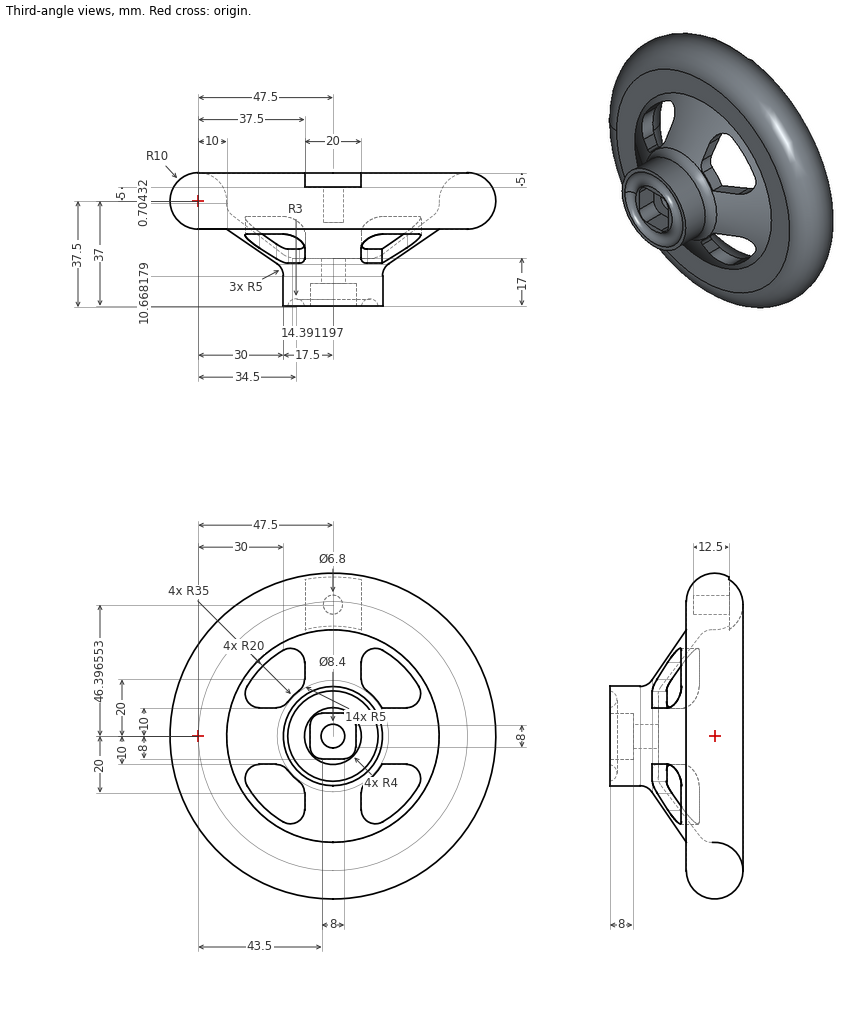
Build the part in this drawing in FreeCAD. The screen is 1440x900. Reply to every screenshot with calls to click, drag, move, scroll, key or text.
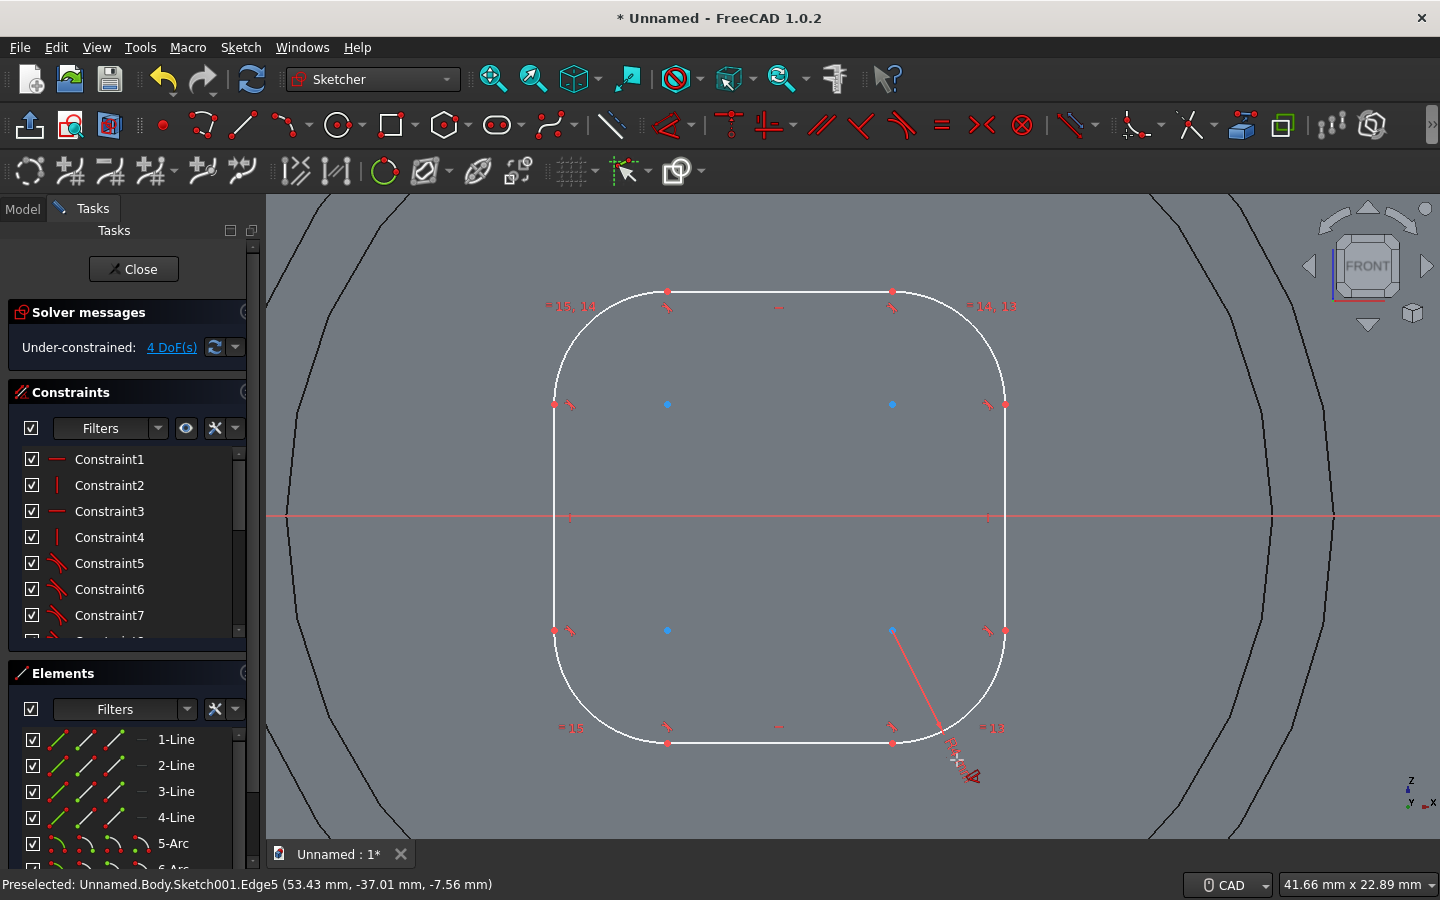
click(735, 743)
click(780, 777)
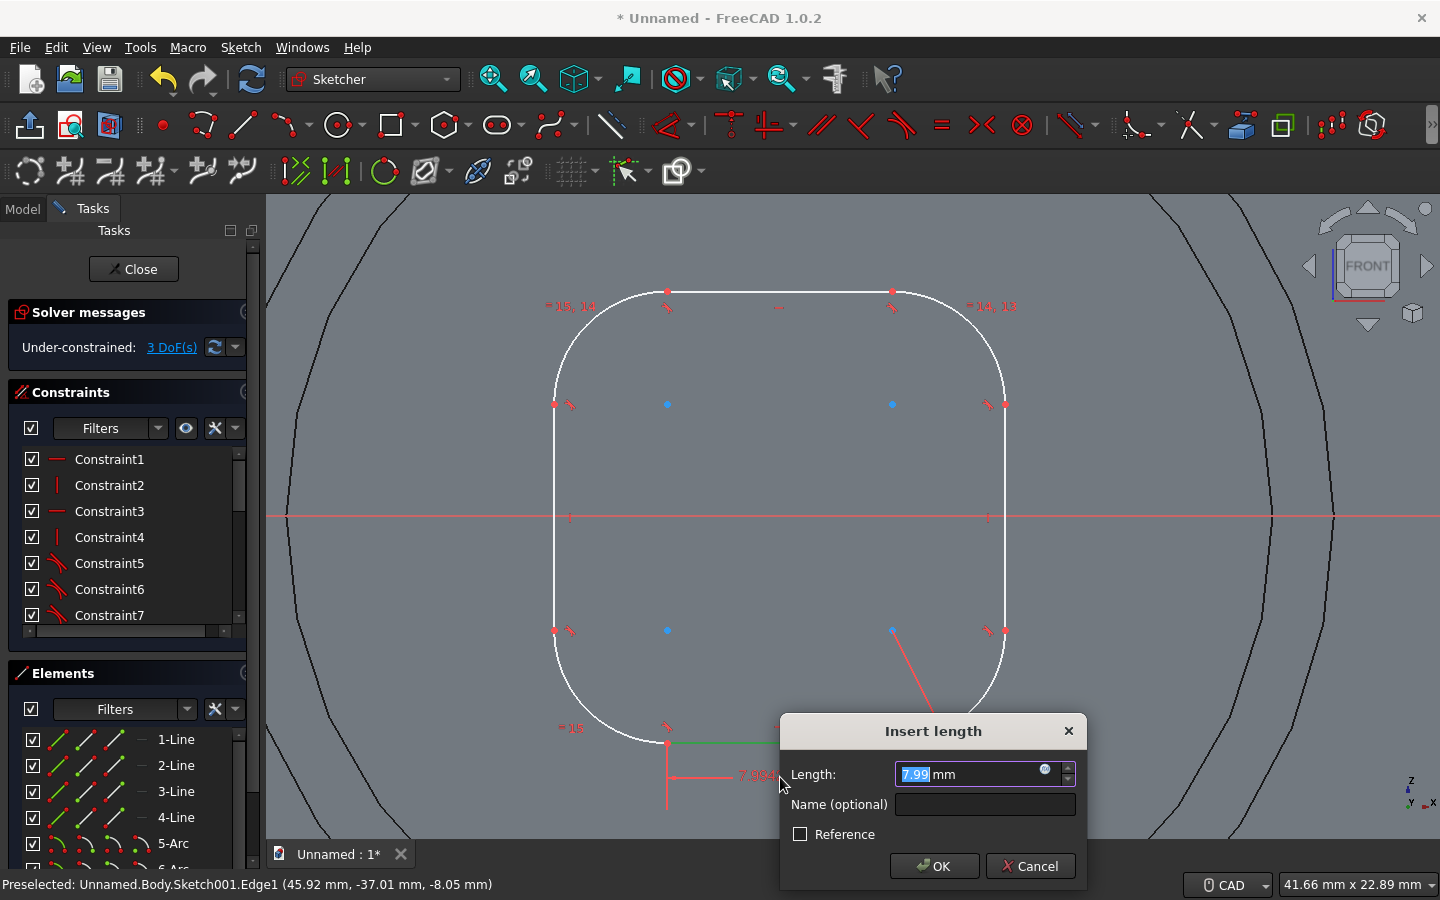
text(8)
key(Return)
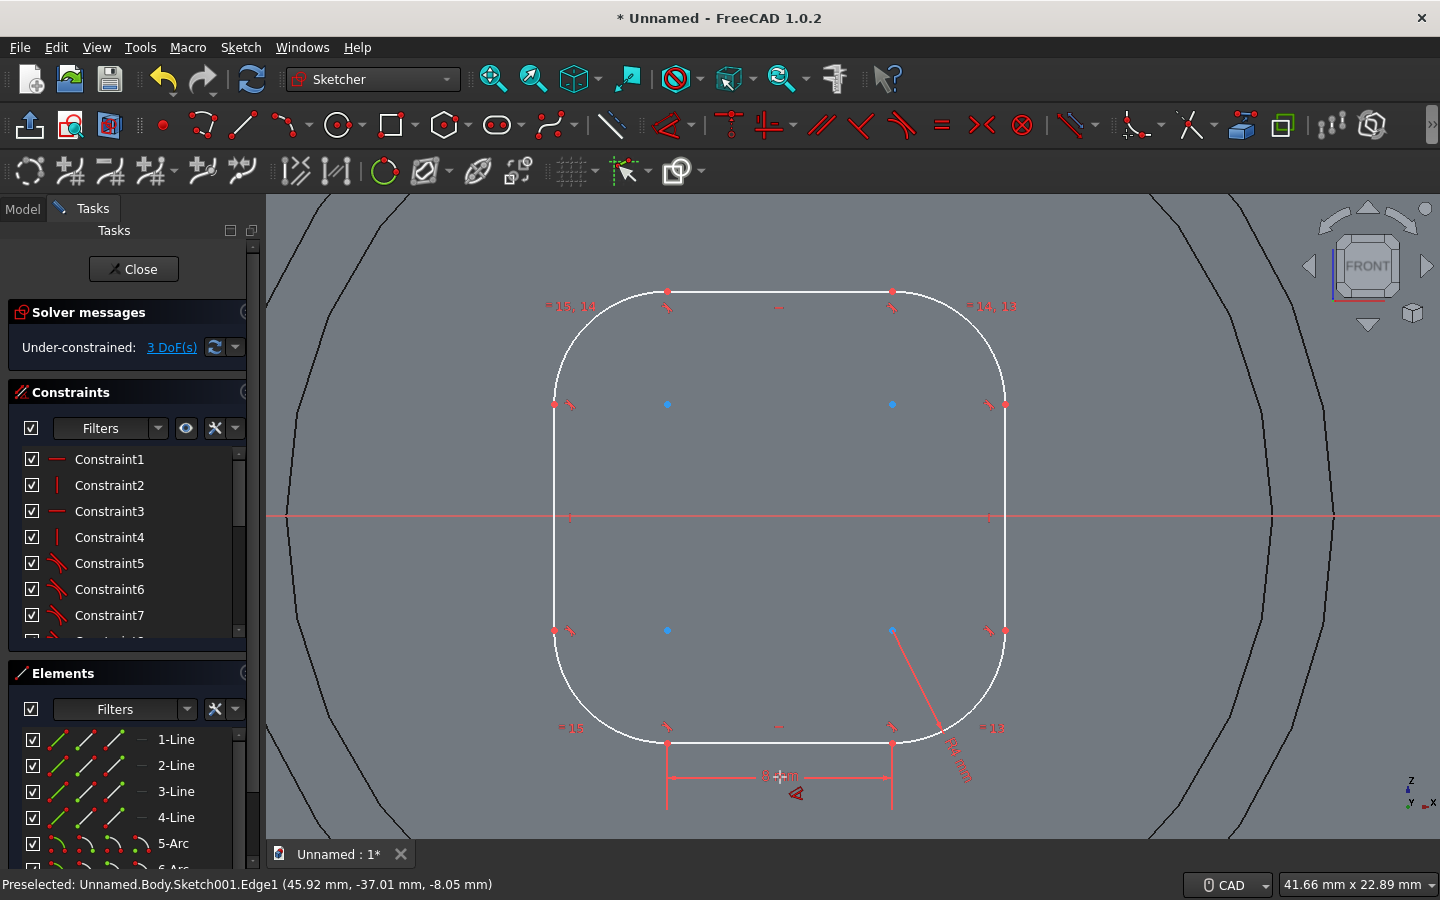
click(1005, 563)
click(1039, 465)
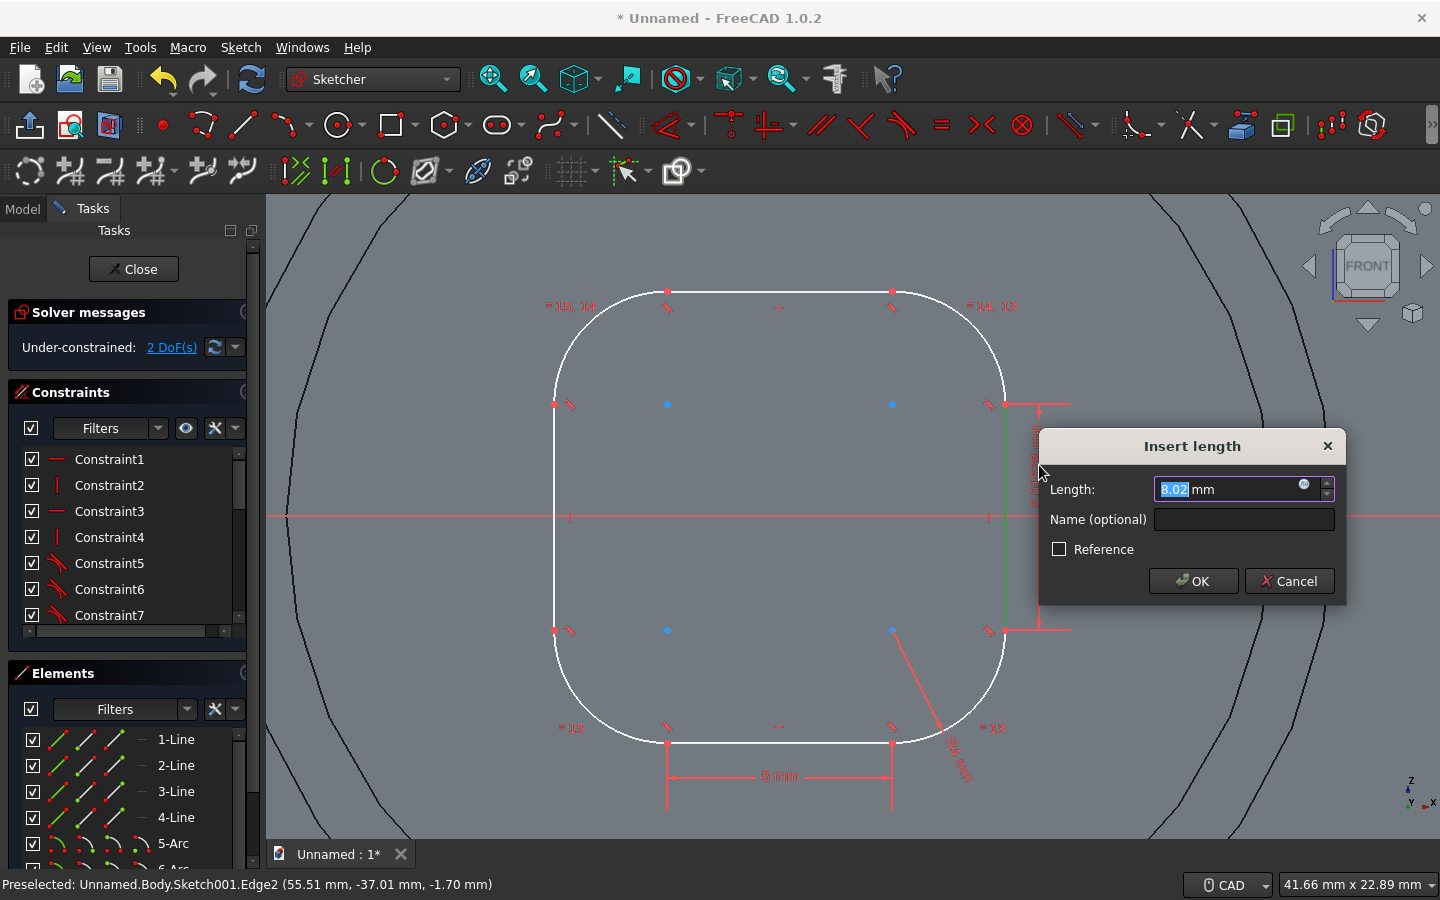
text(8)
key(Return)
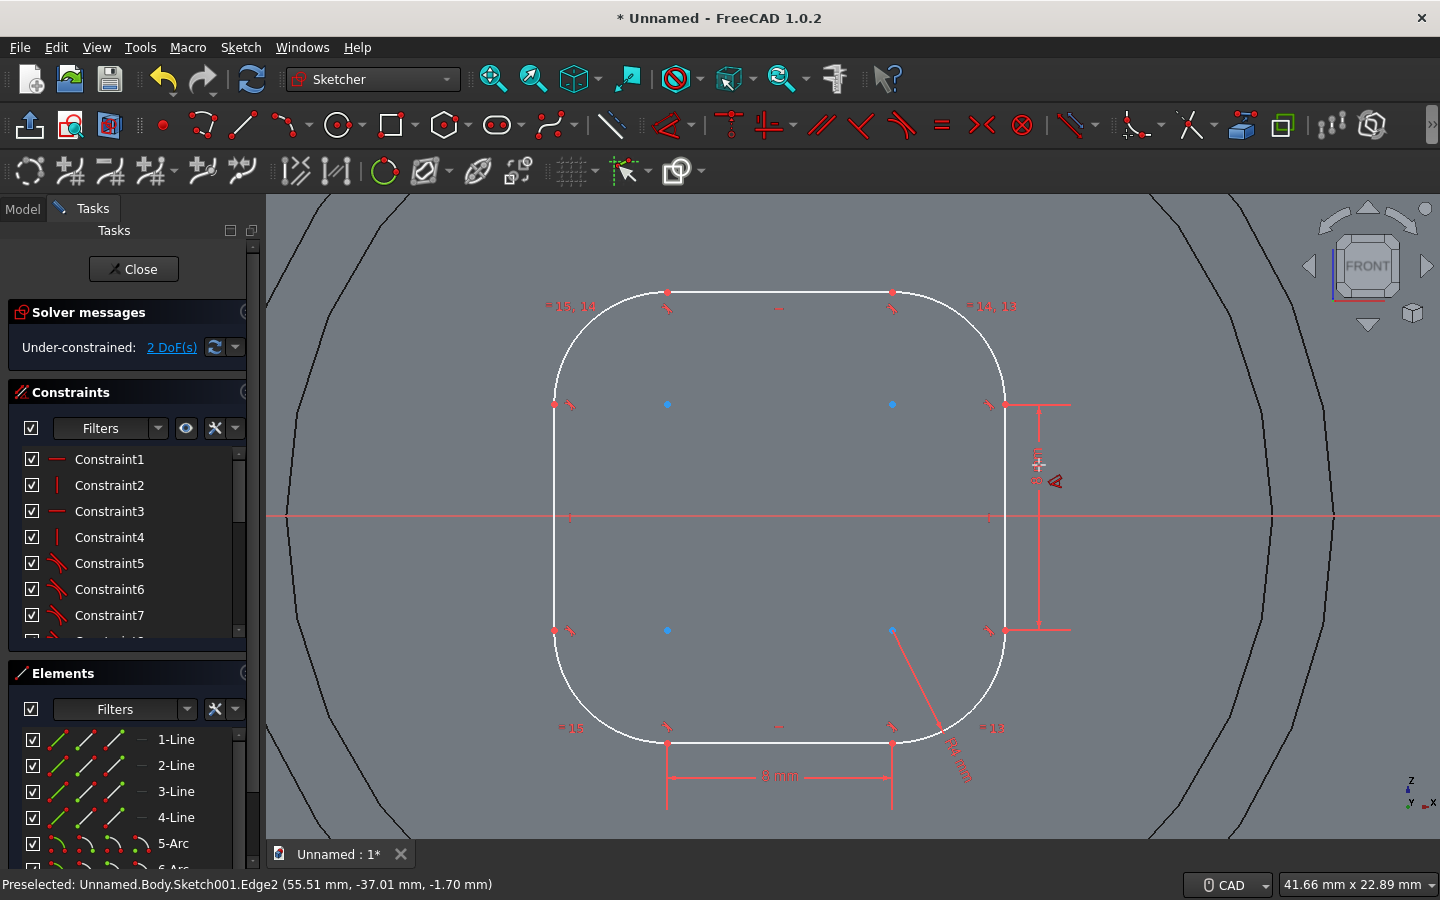
click(667, 743)
click(701, 630)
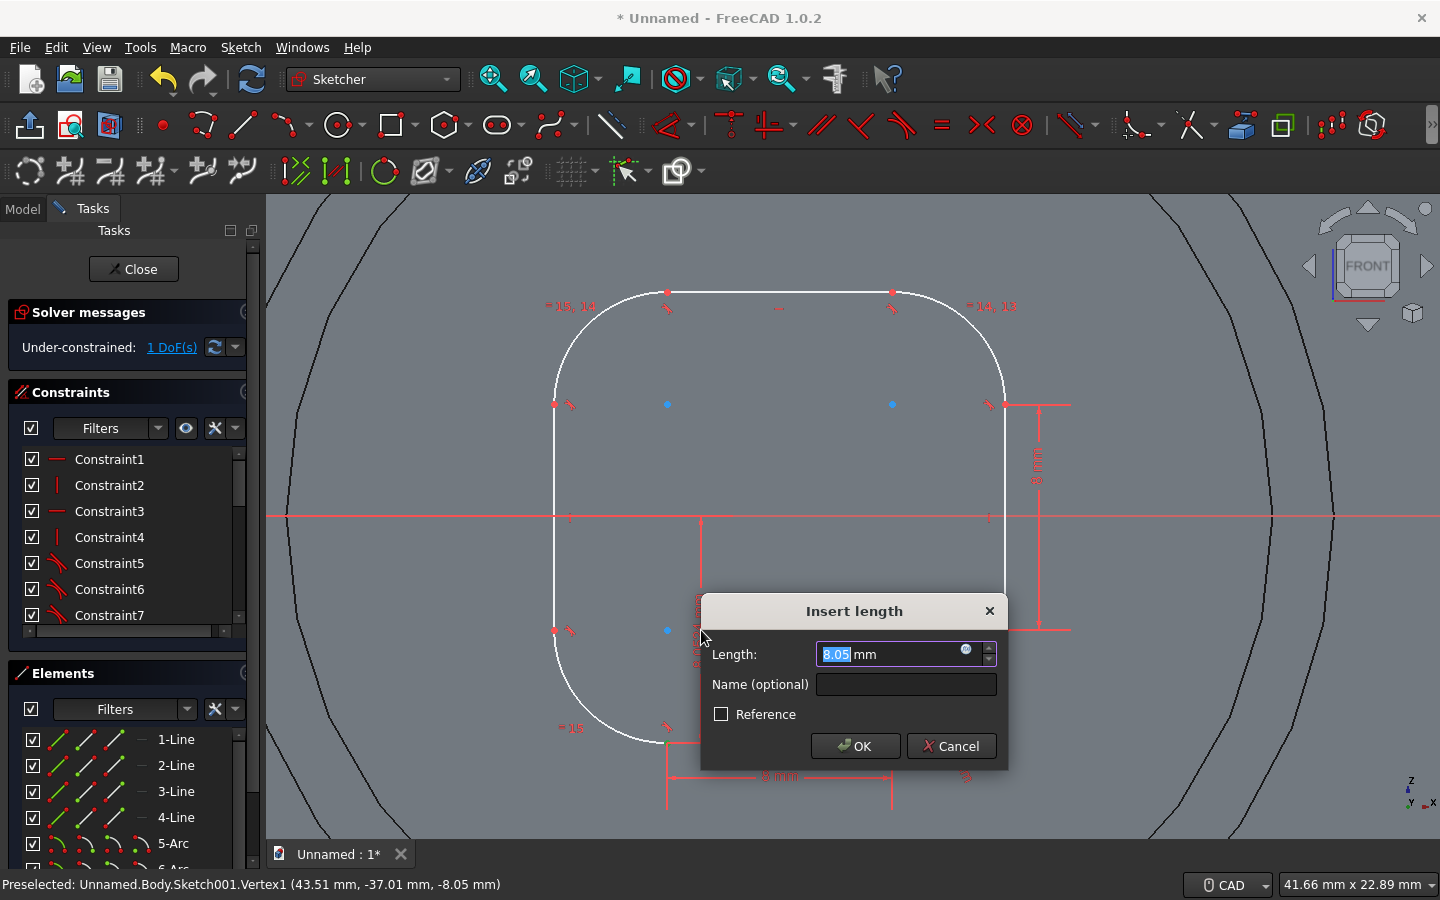
text(8)
key(Return)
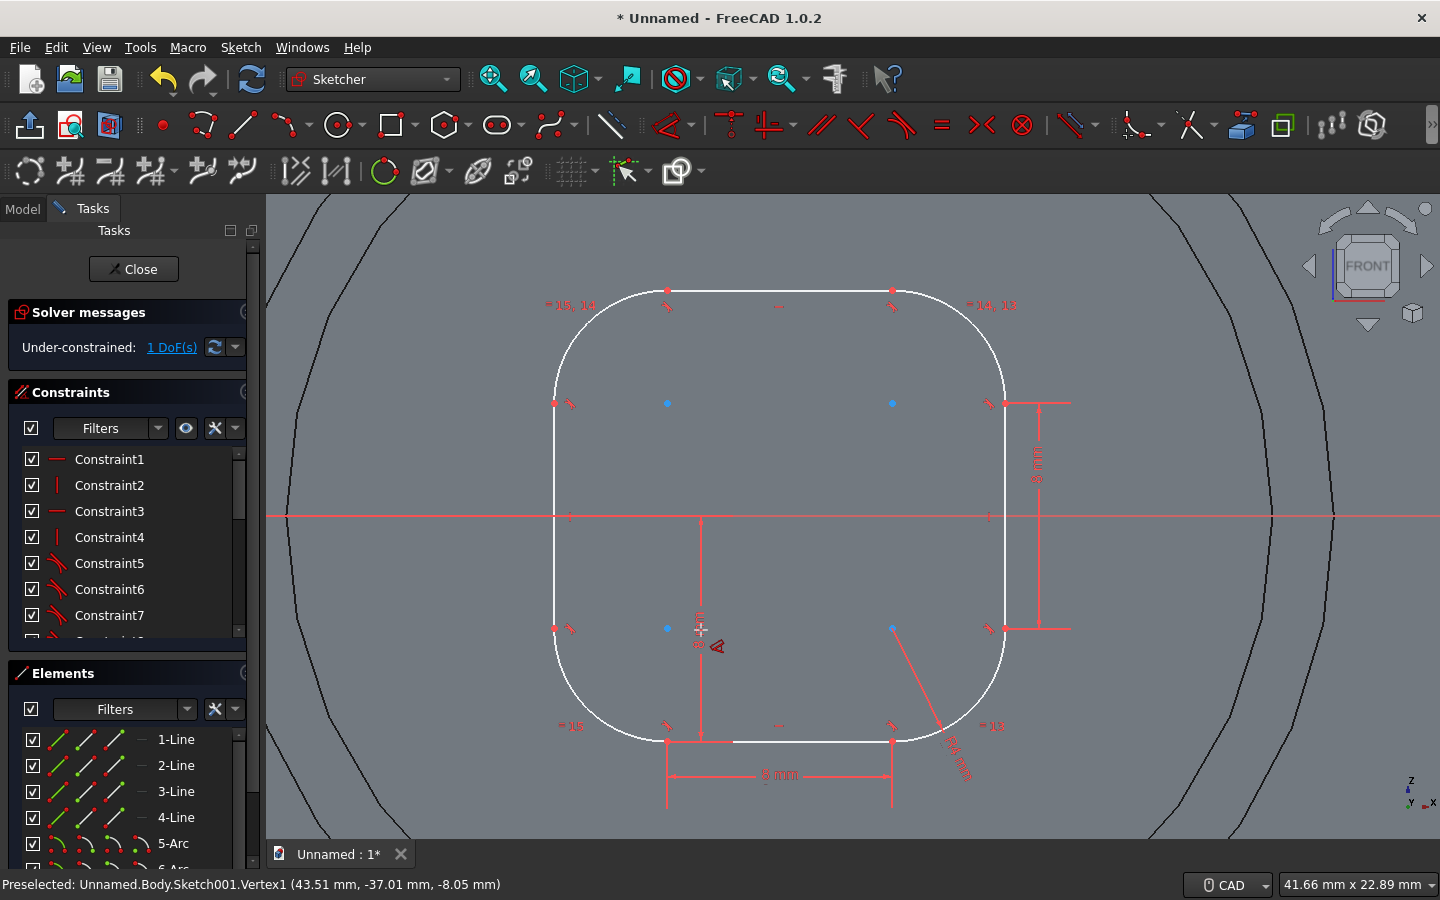
click(667, 742)
click(481, 776)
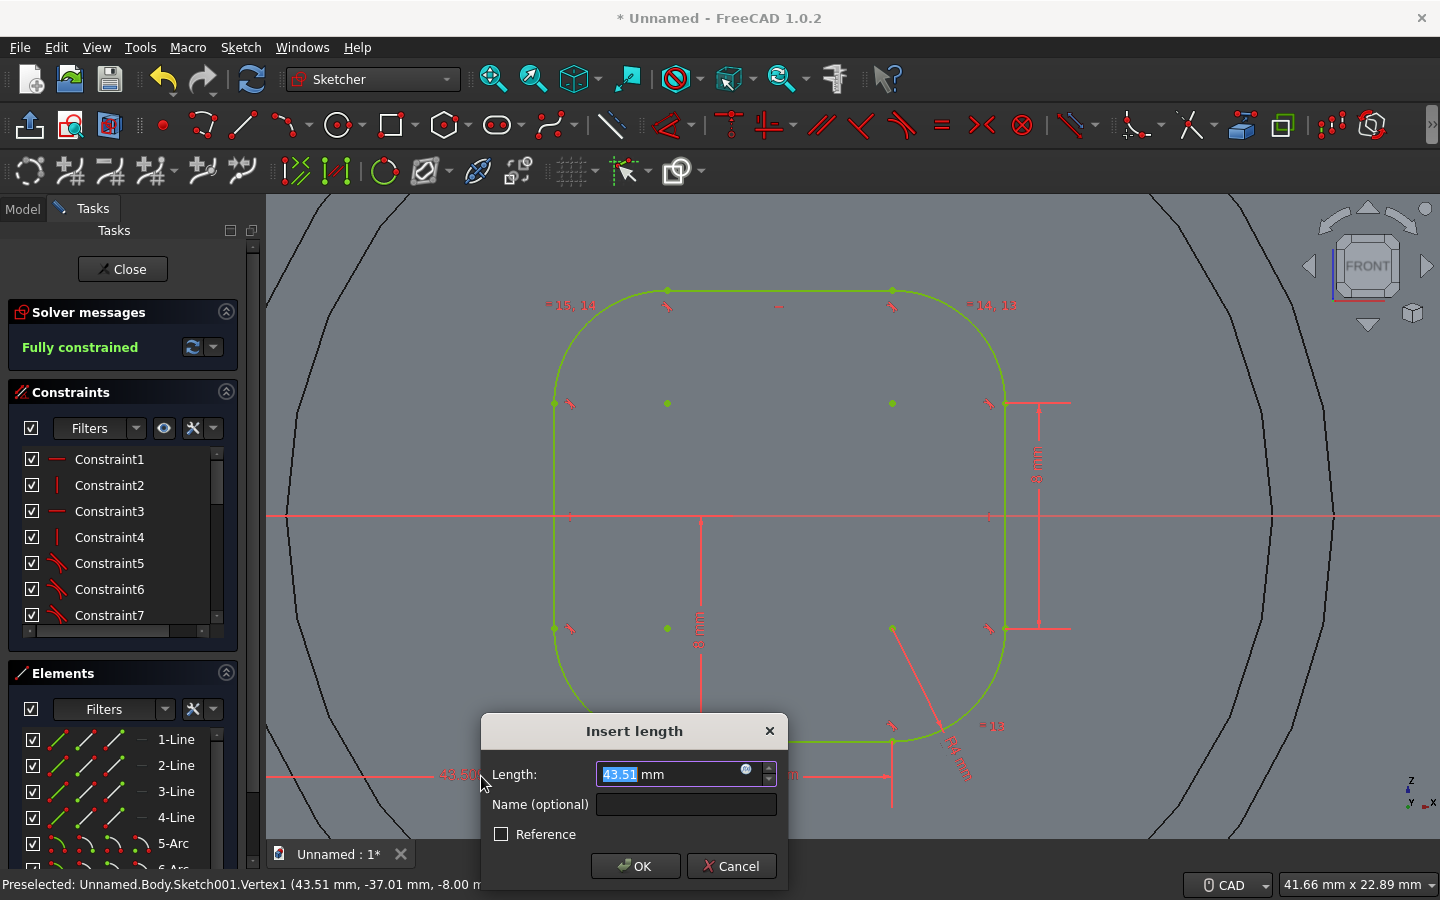
text(43.5)
key(Return)
key(Escape)